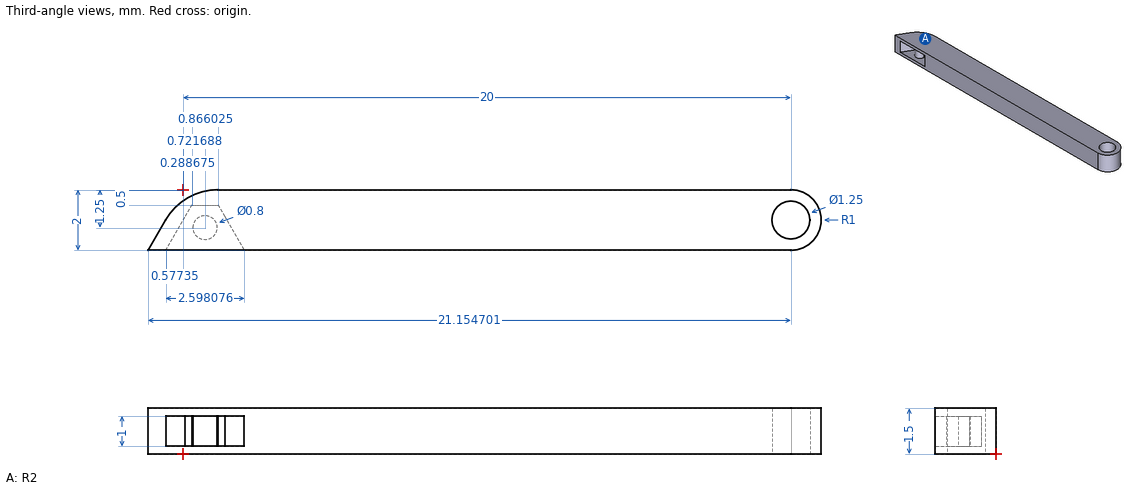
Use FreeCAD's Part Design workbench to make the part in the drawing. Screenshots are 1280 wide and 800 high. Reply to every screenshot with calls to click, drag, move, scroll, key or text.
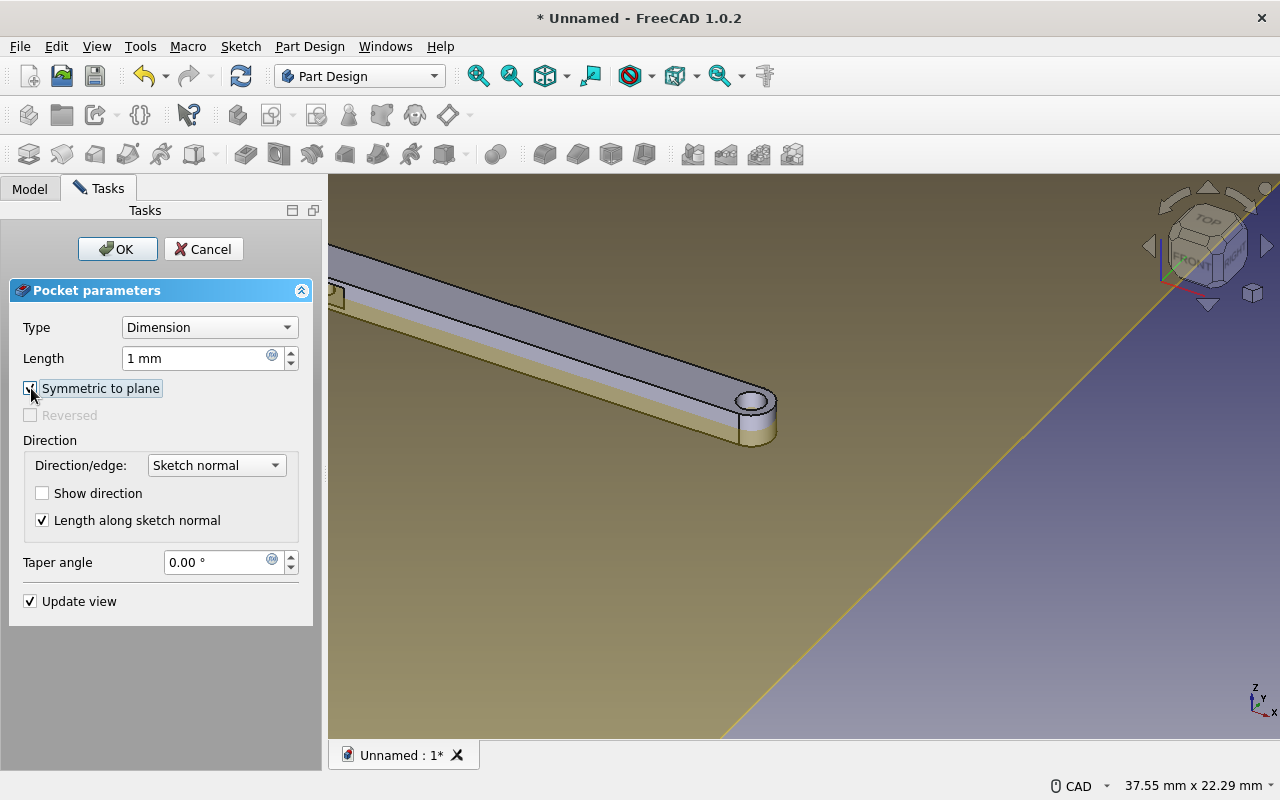
click(118, 249)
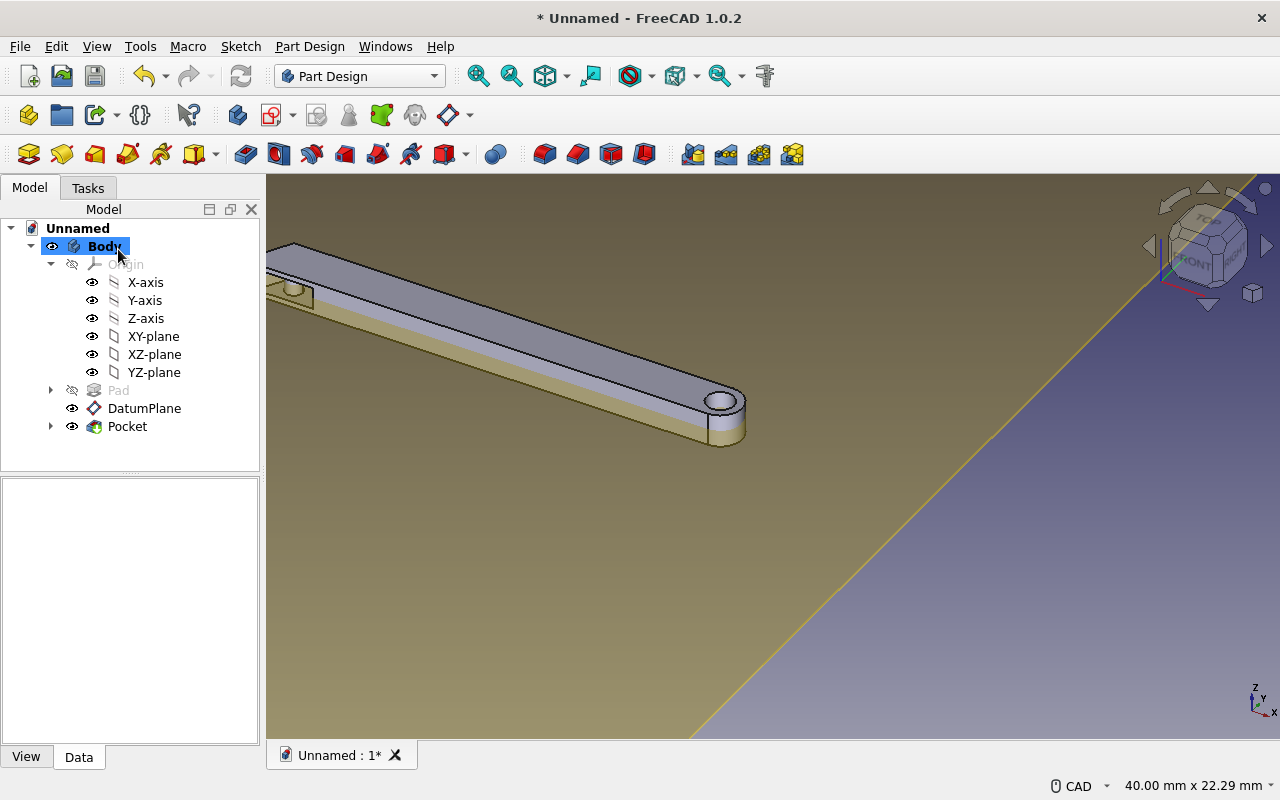
click(117, 408)
key(space)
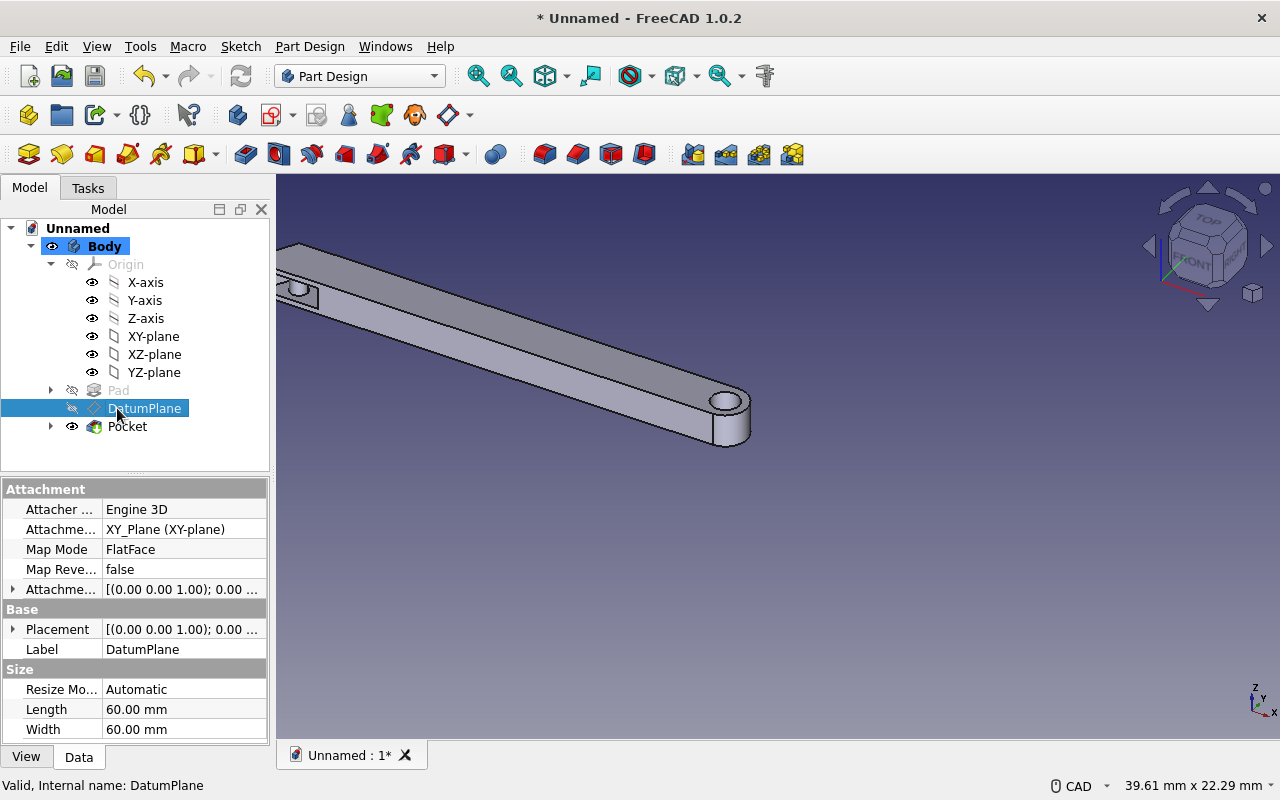
key(v)
key(f)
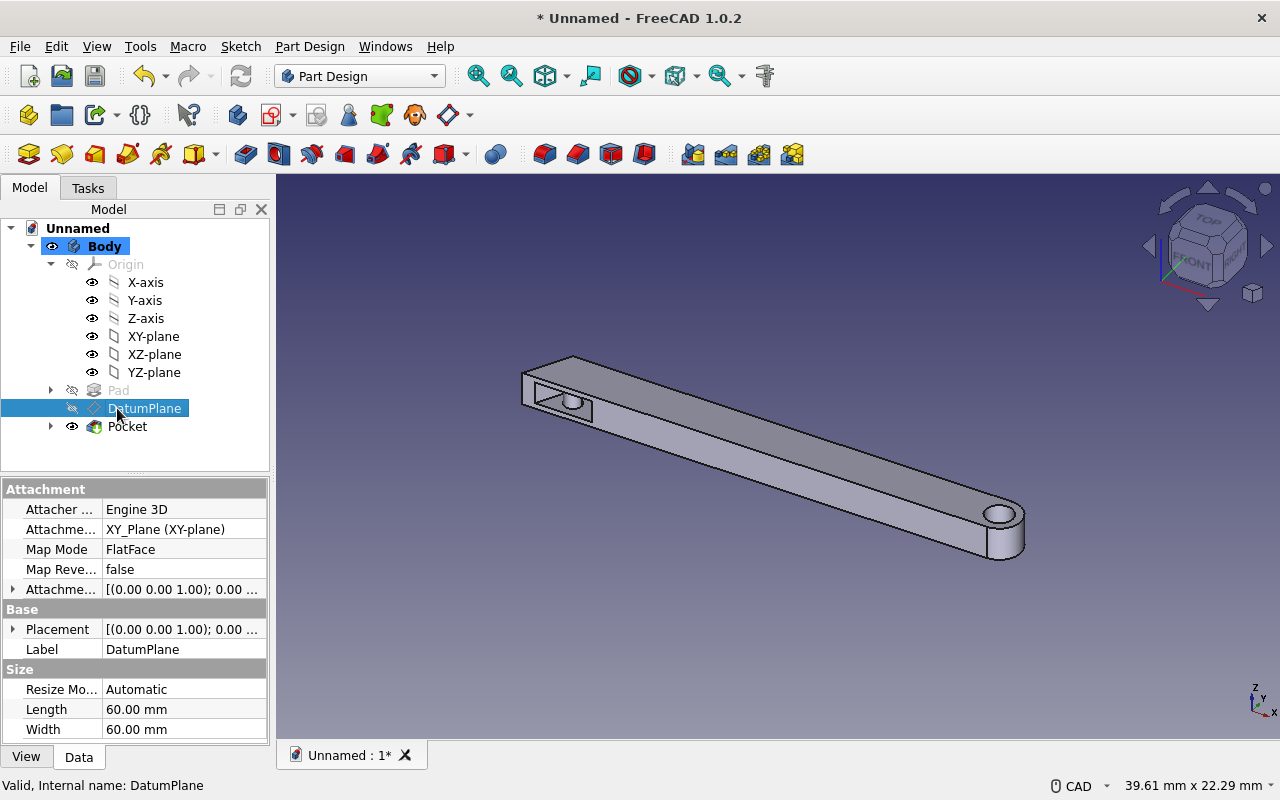
key(0)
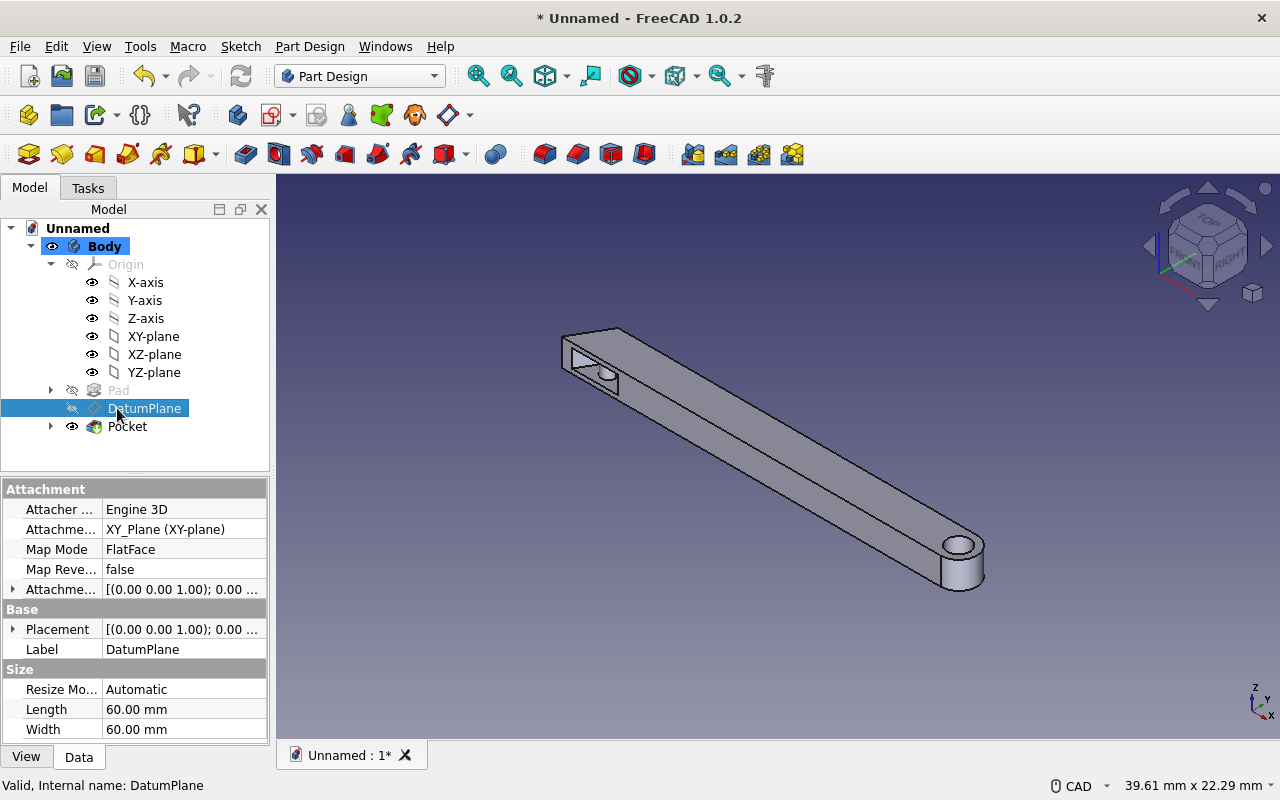
key(2)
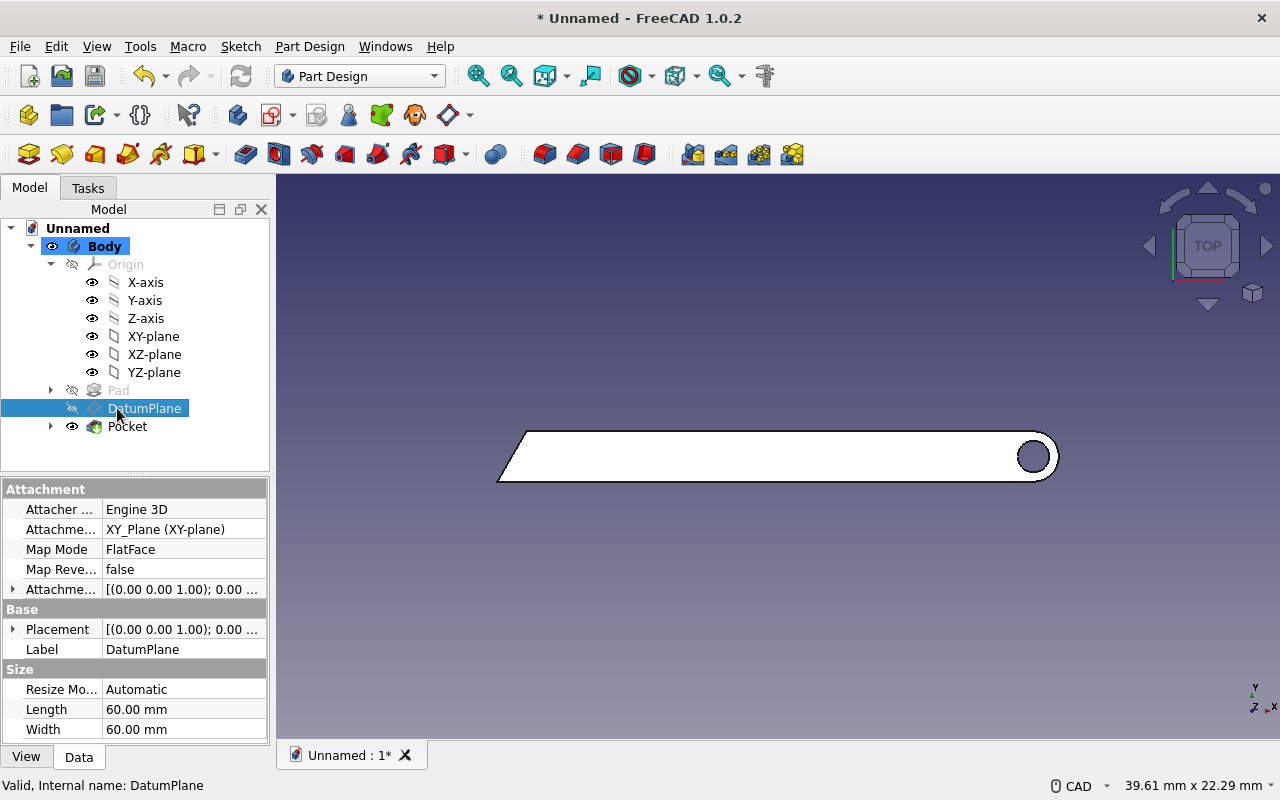
key(1)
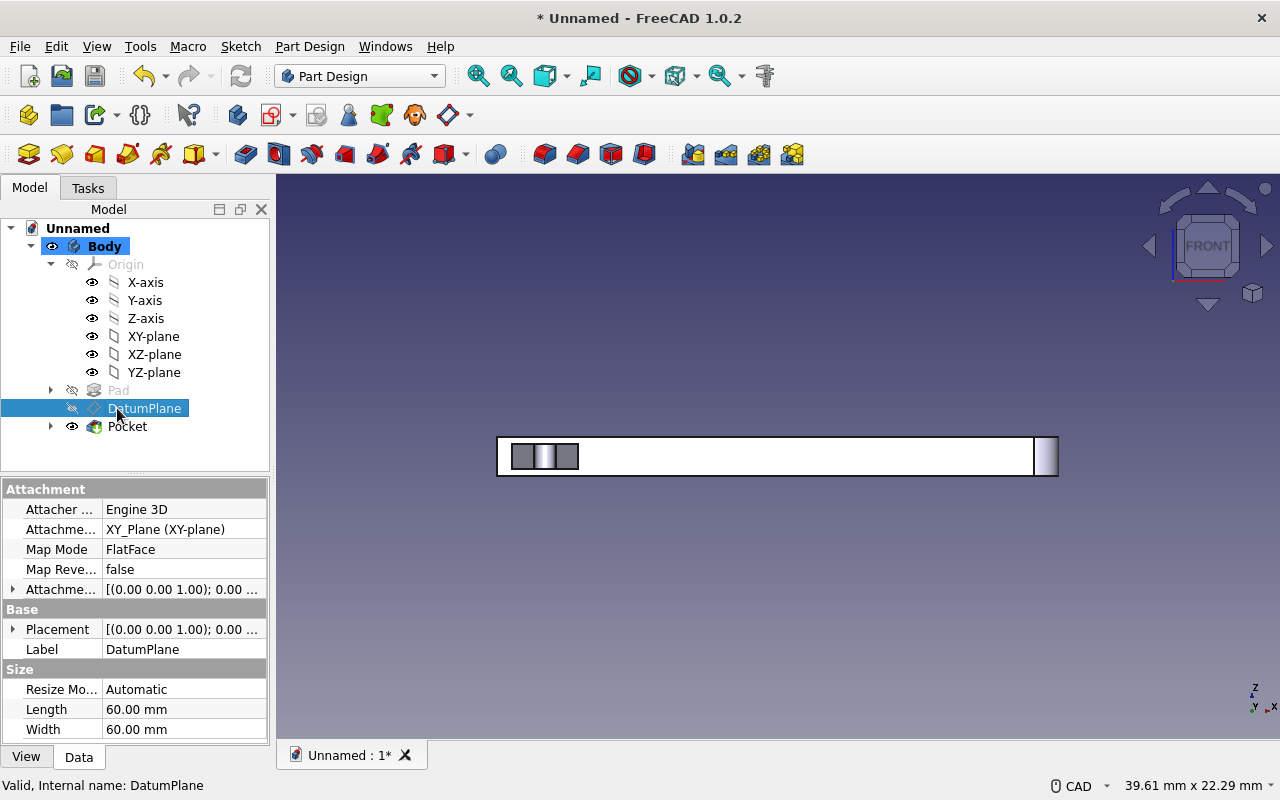
key(3)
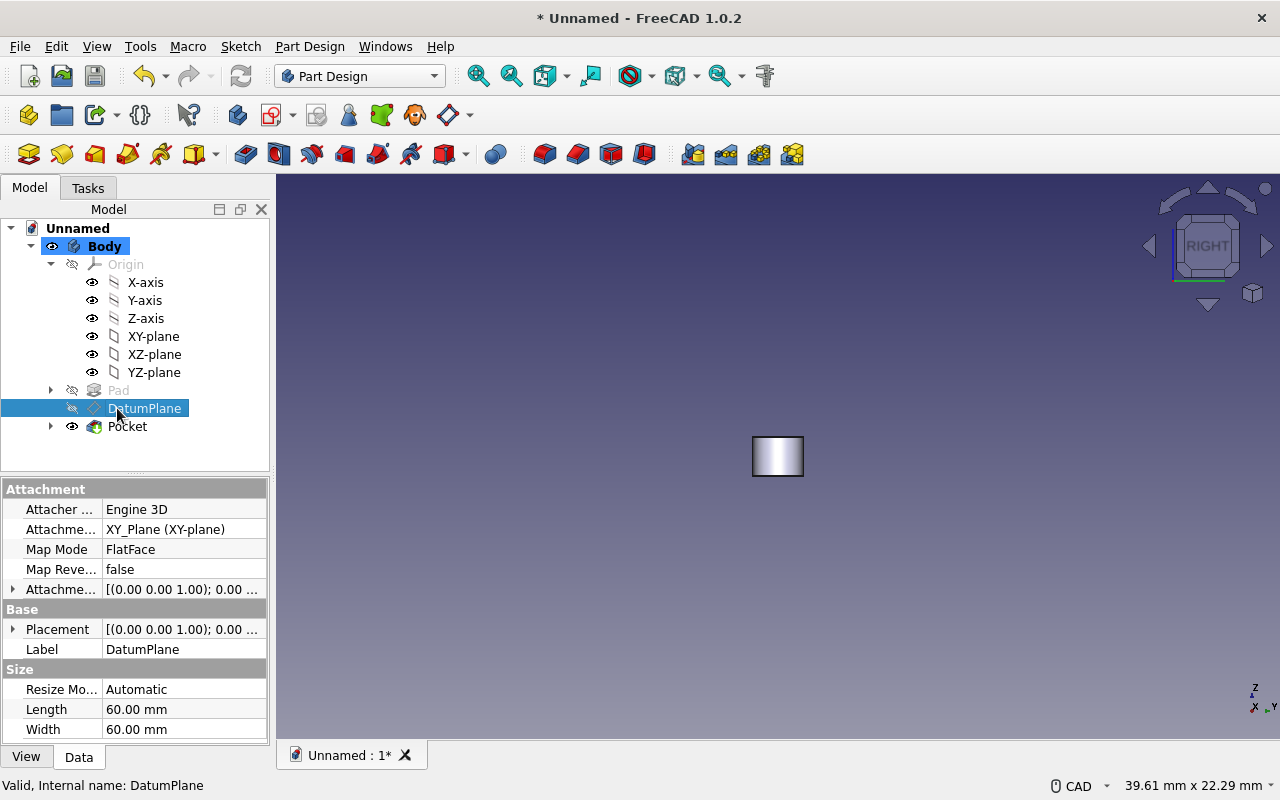
click(479, 76)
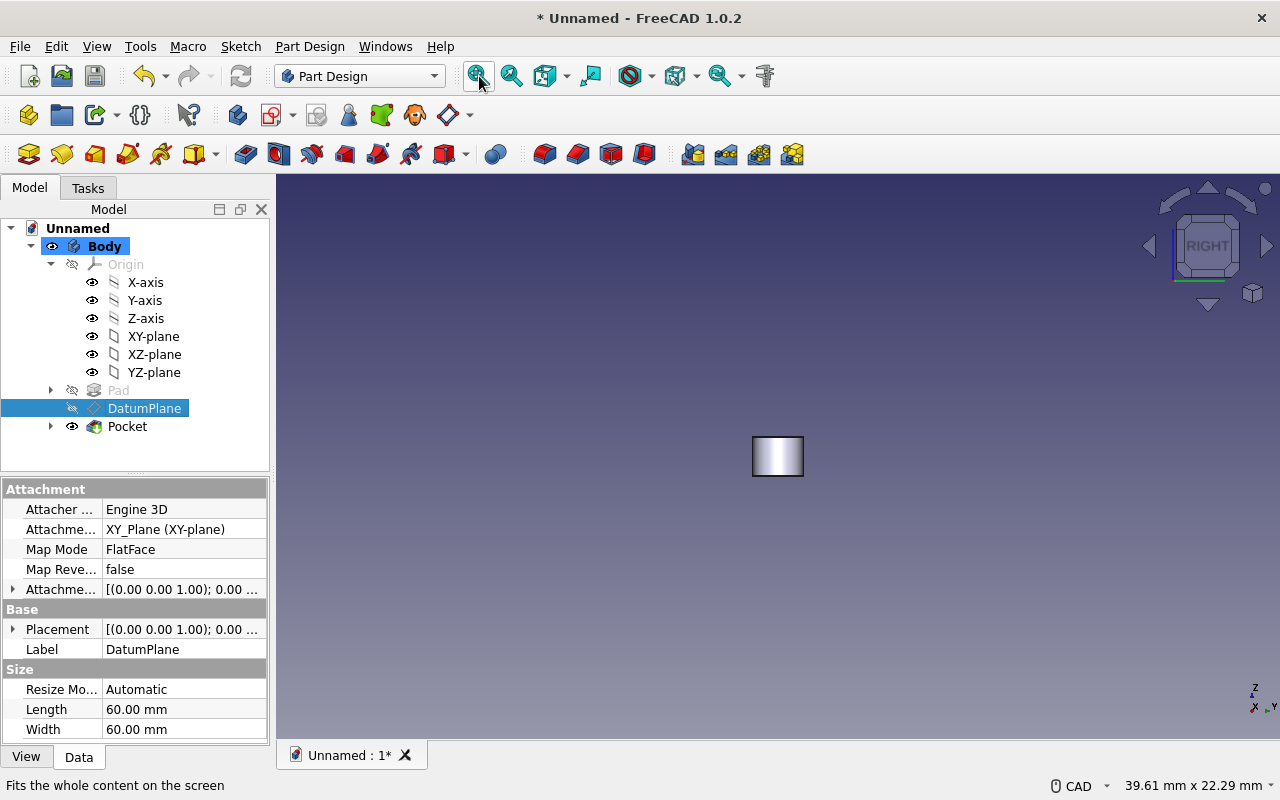
key(5)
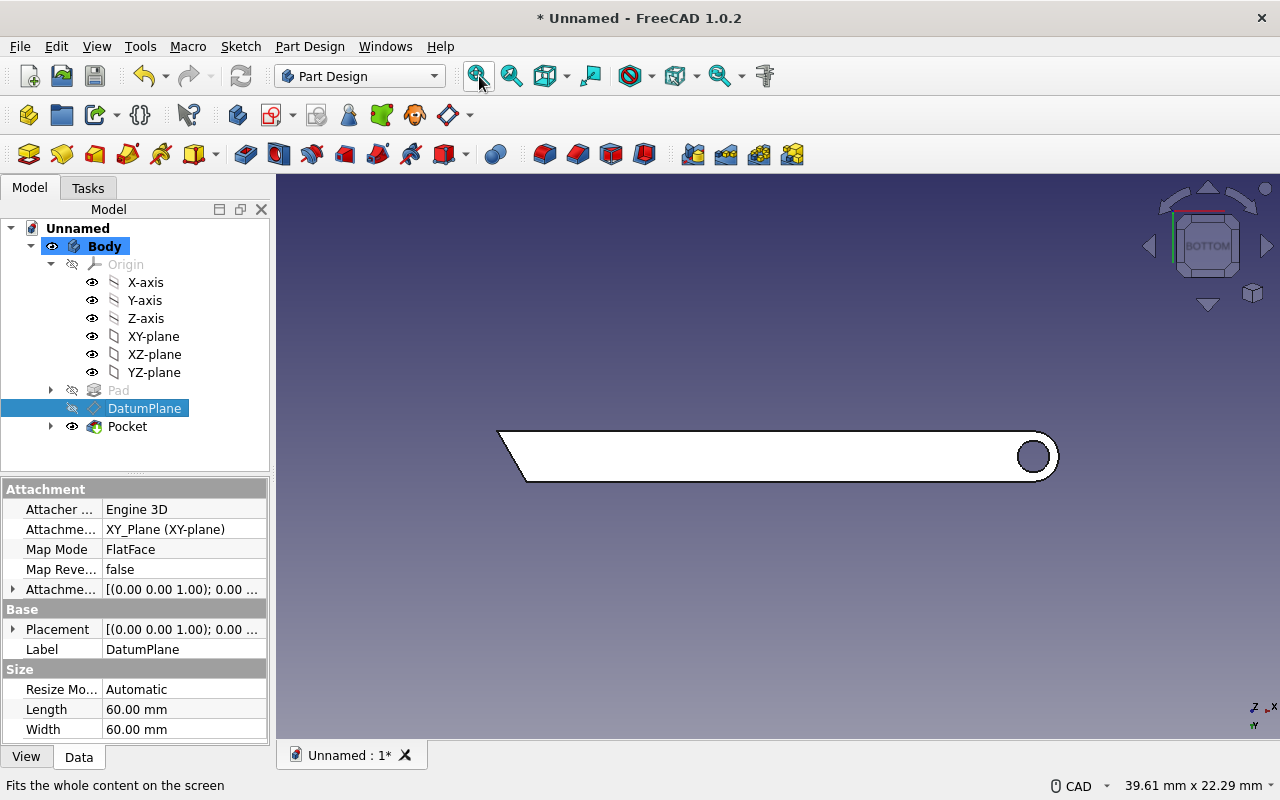
key(4)